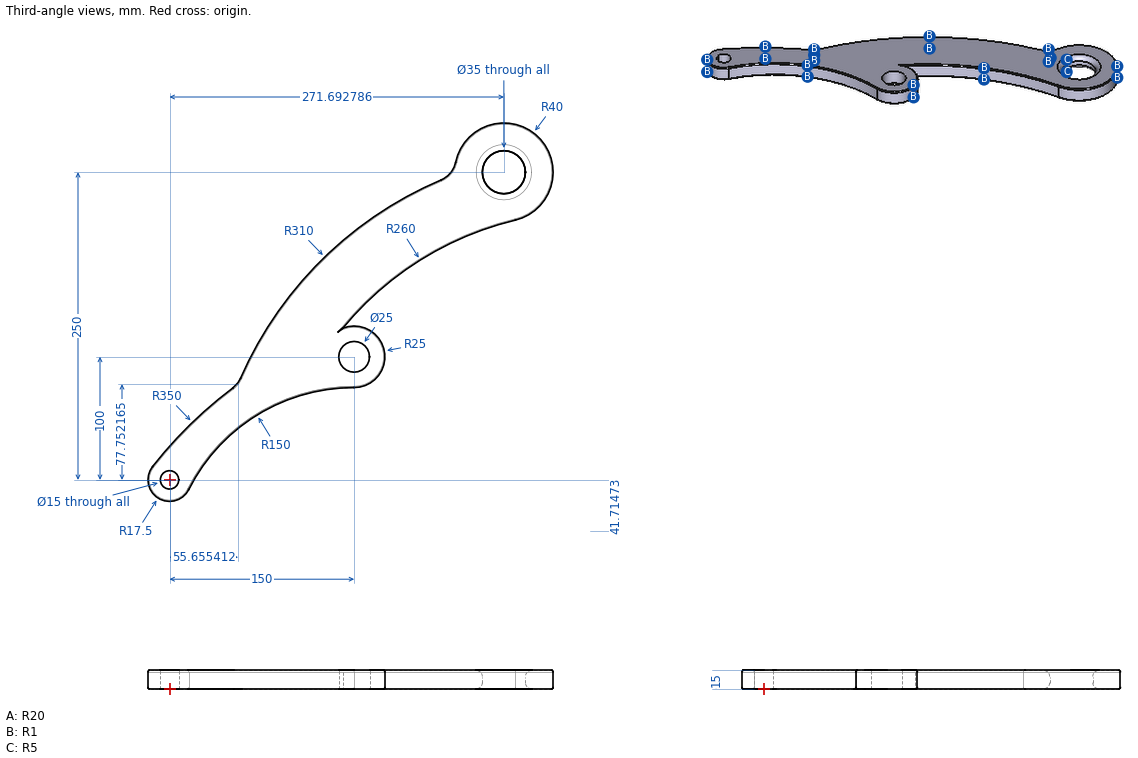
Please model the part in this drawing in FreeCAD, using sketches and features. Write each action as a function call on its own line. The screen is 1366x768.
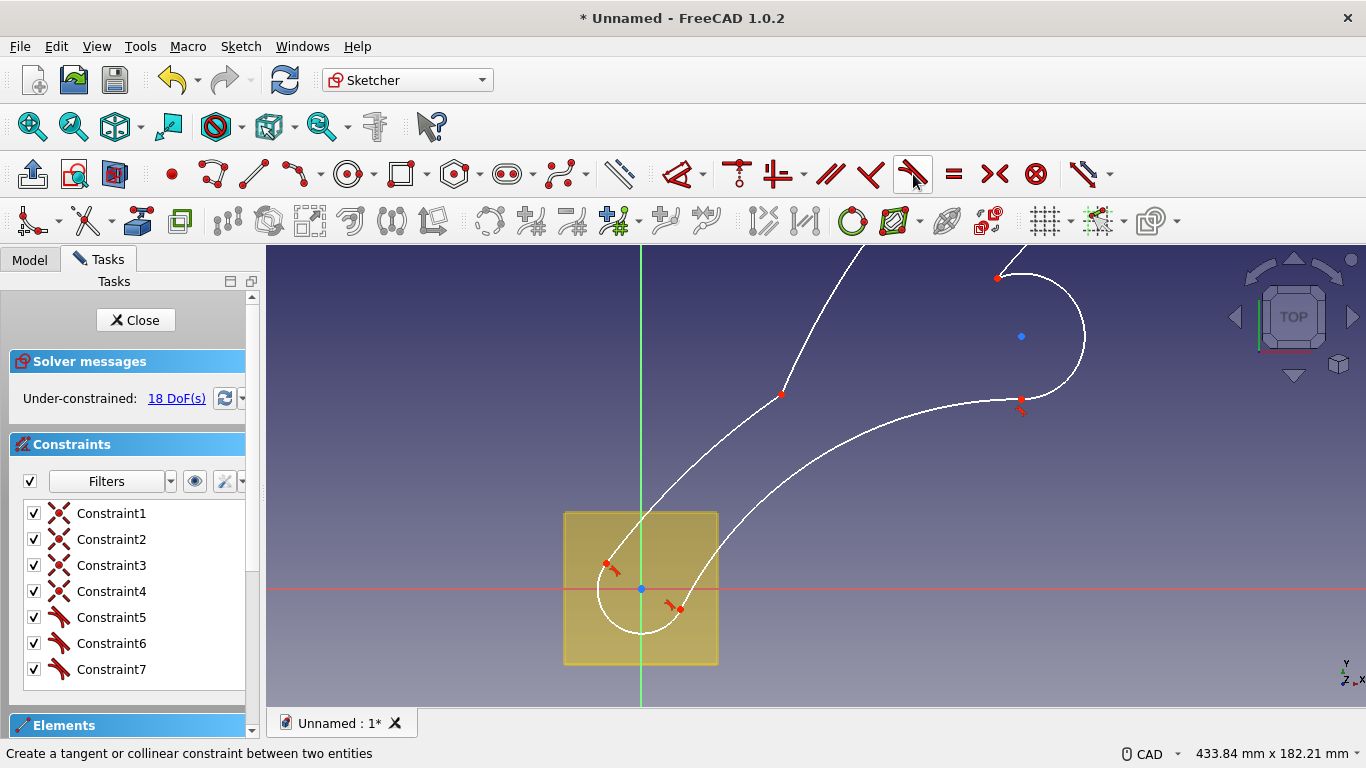
scroll(601, 608, down, 5)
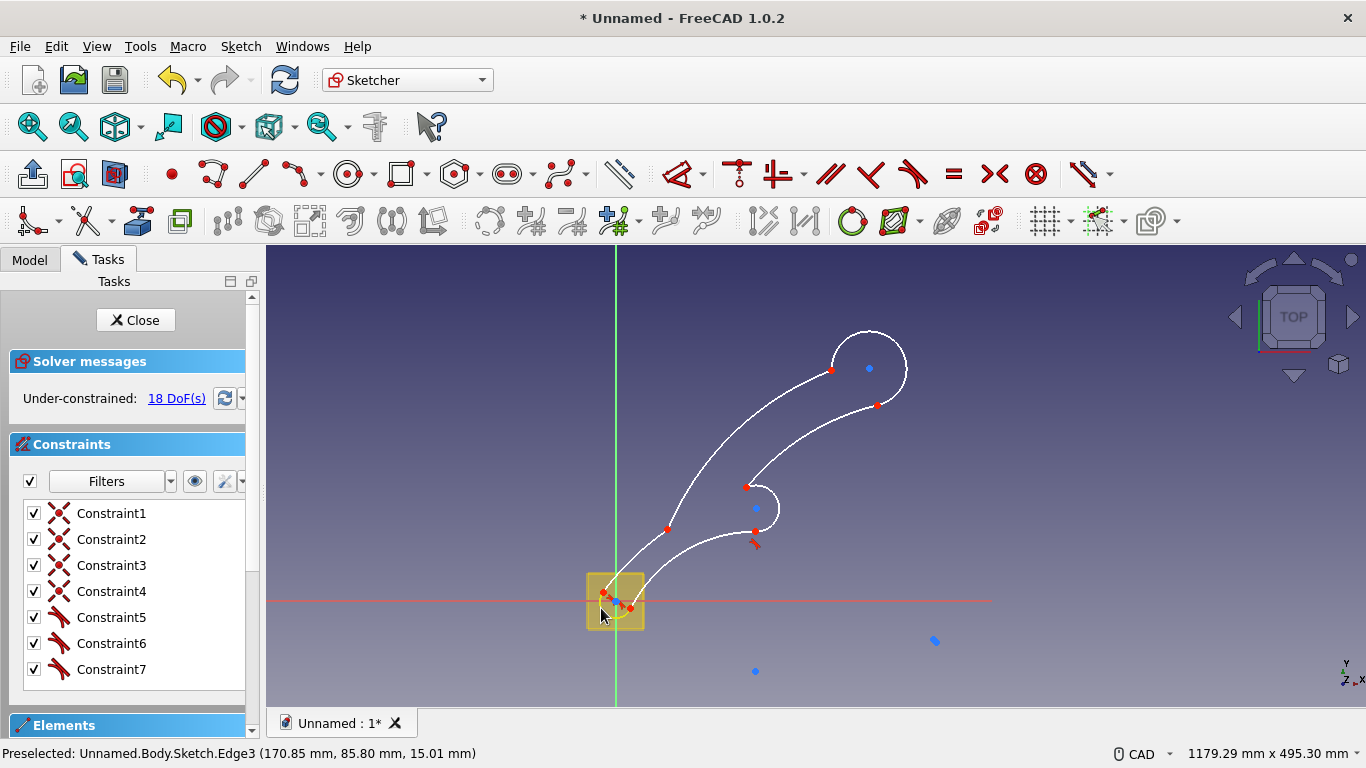
click(833, 421)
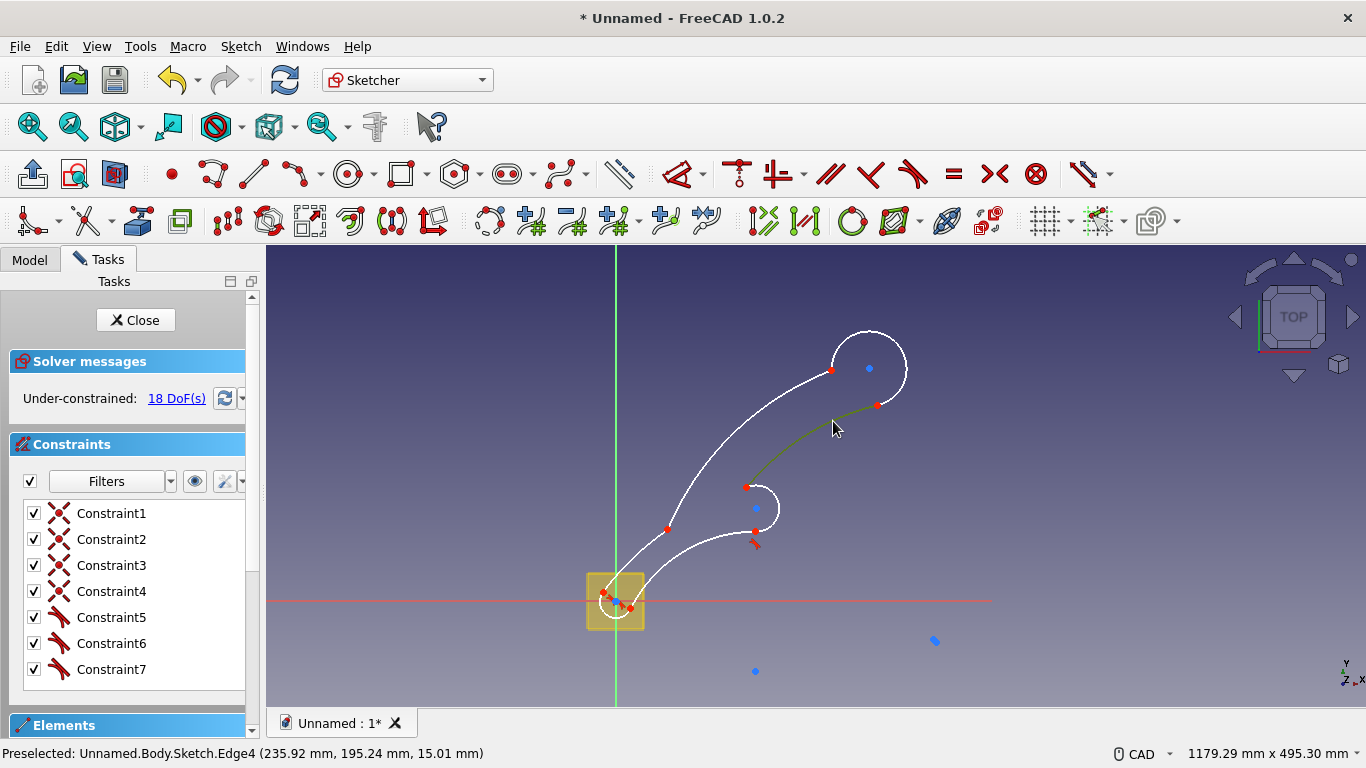
click(907, 368)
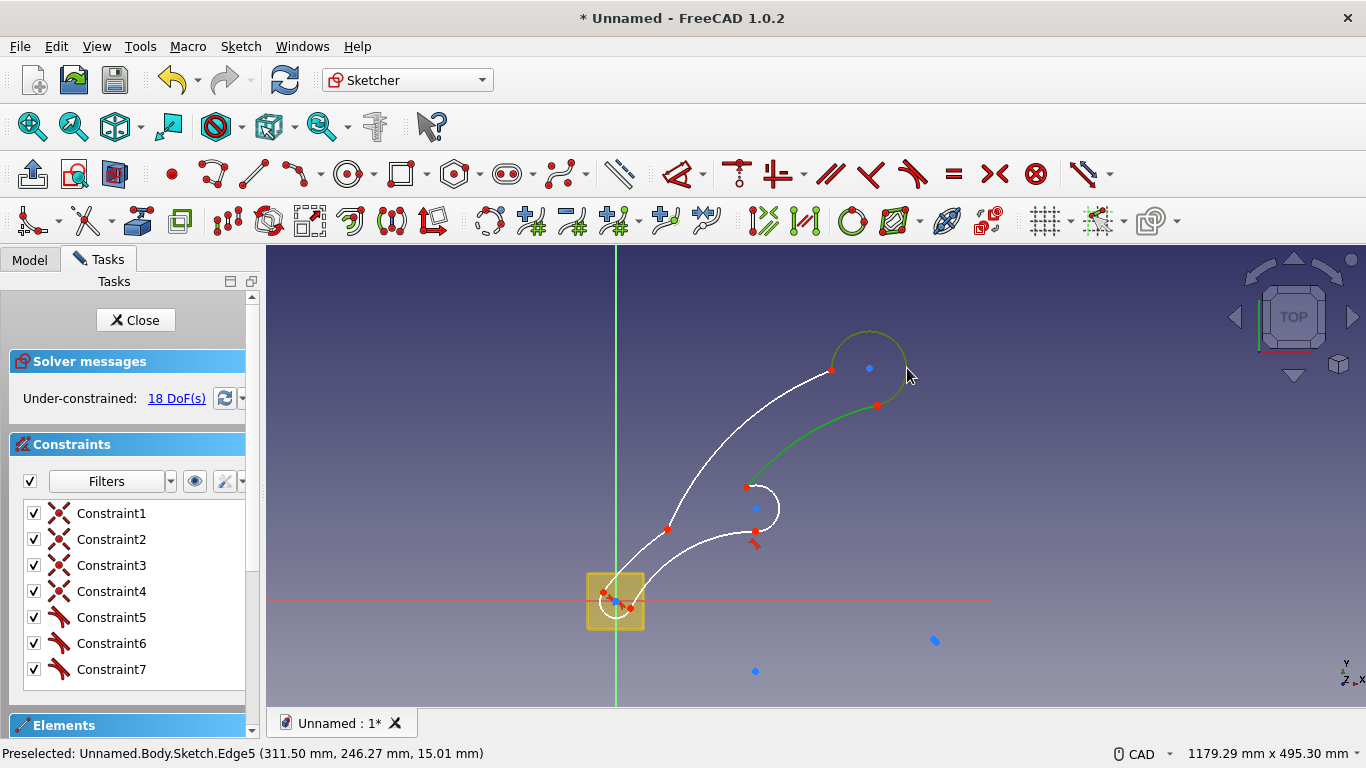
click(913, 174)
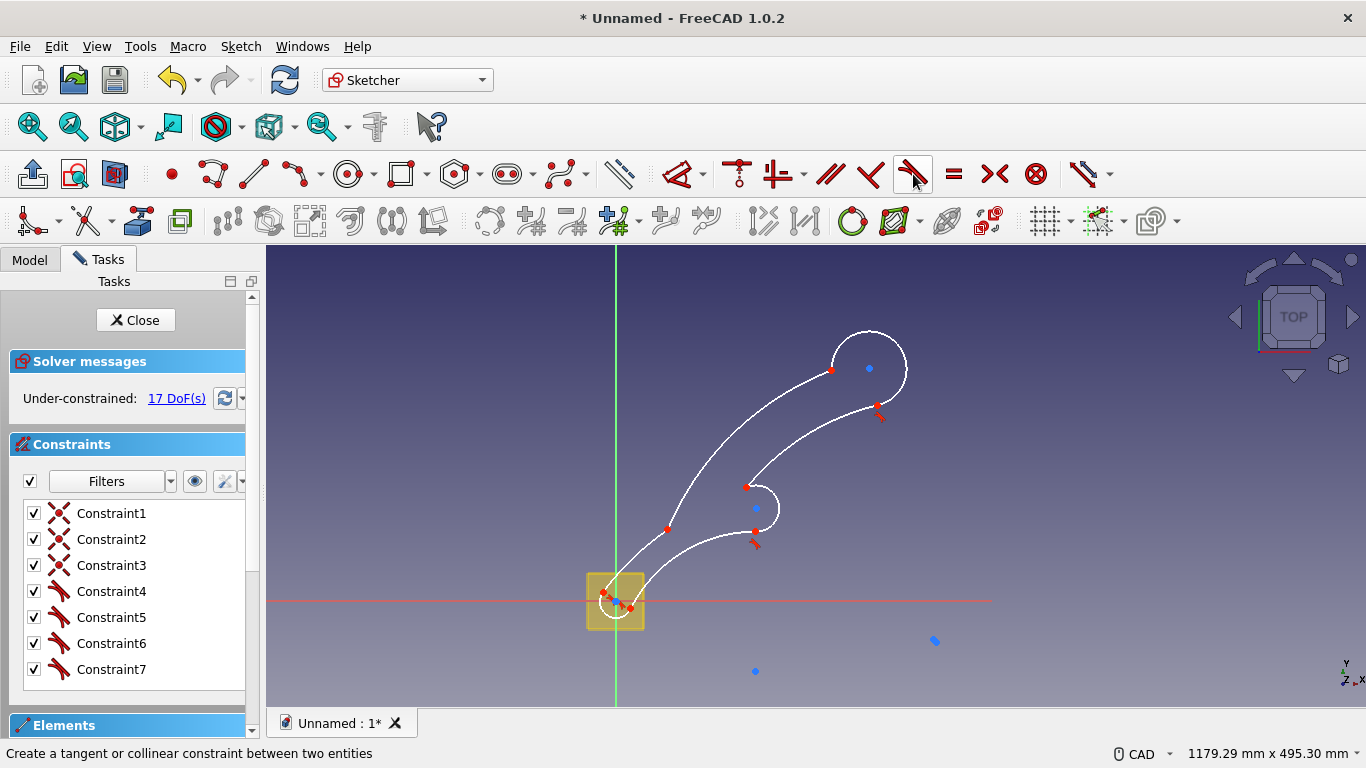
click(833, 421)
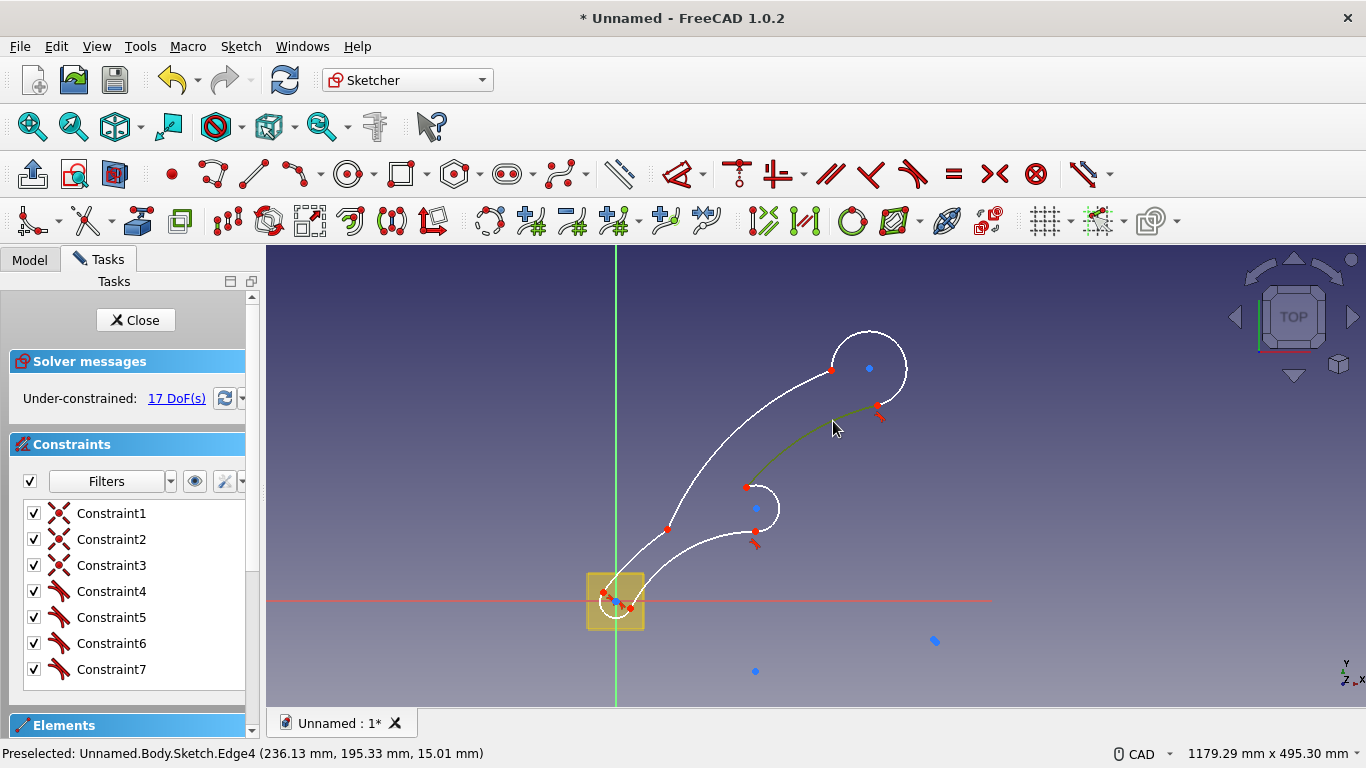
click(770, 403)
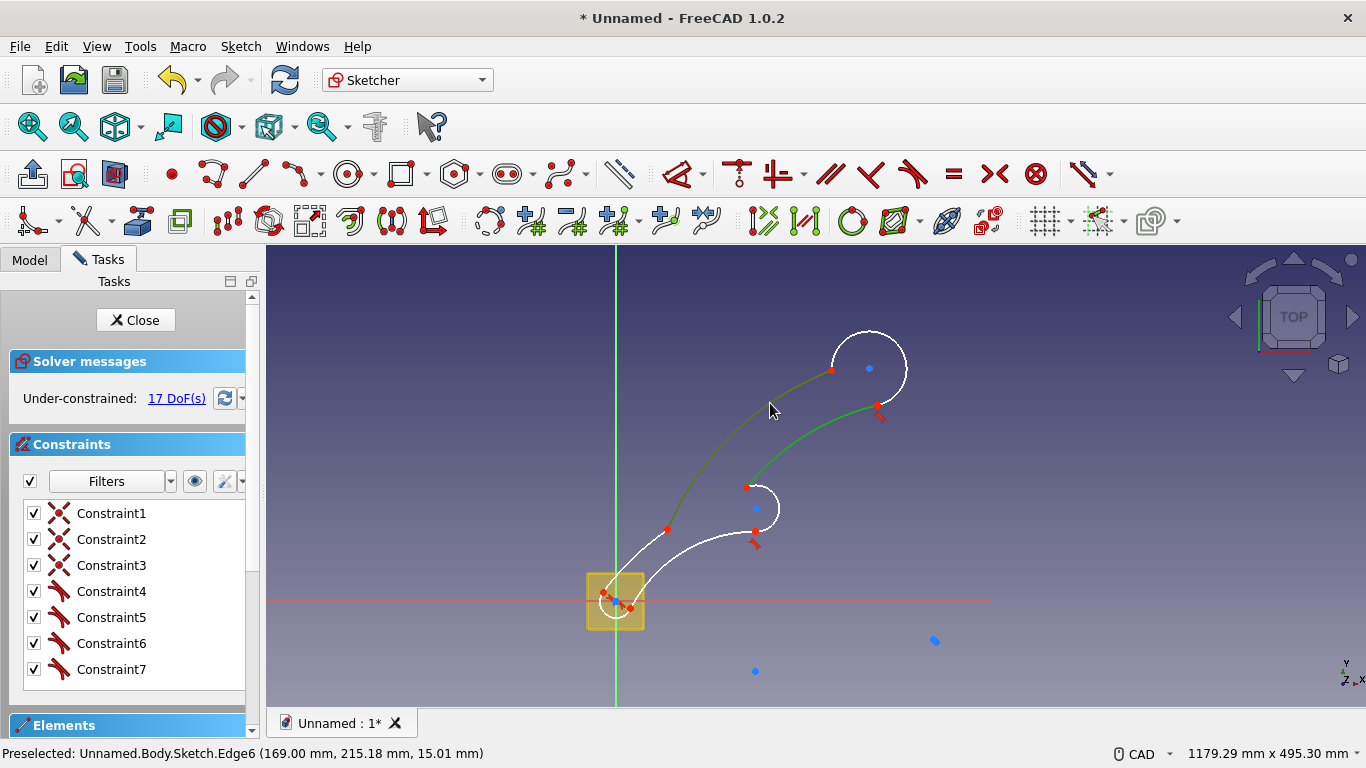
click(737, 174)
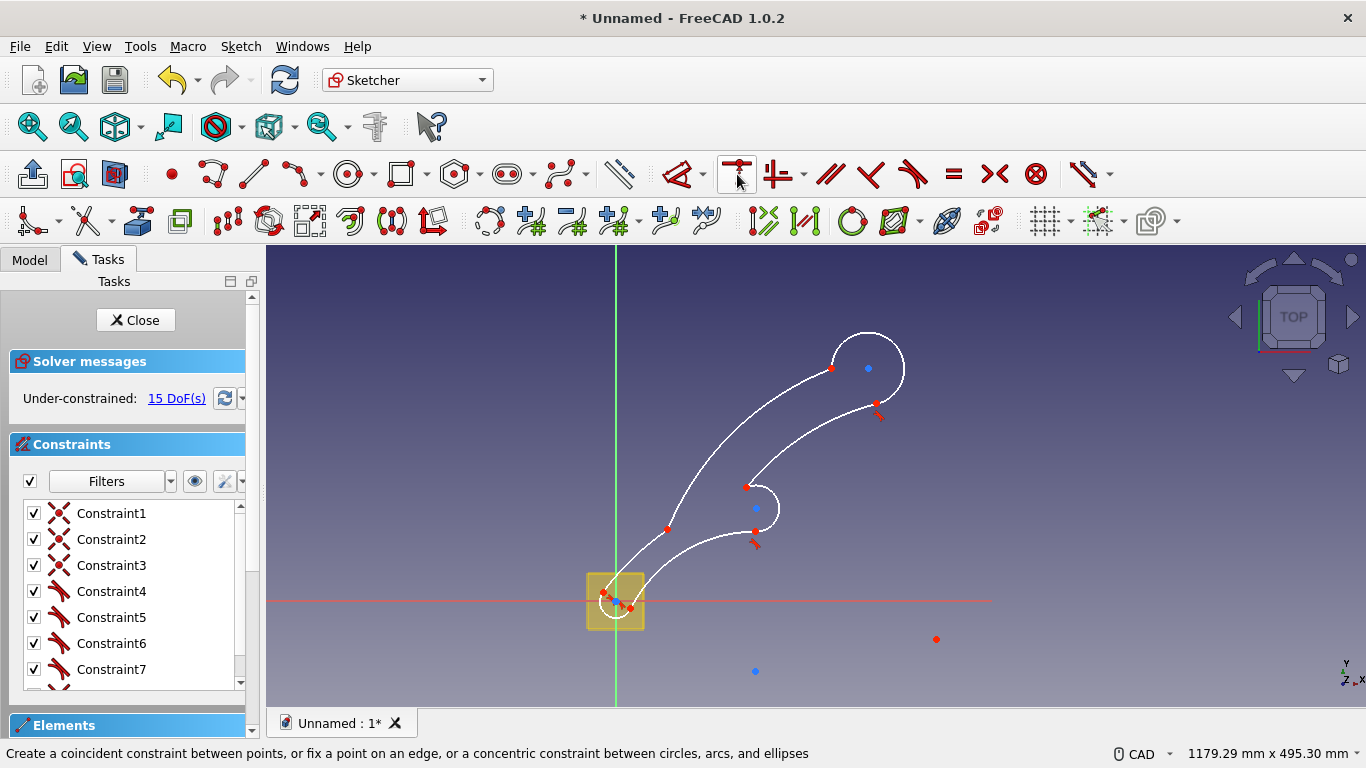
scroll(616, 602, up, 5)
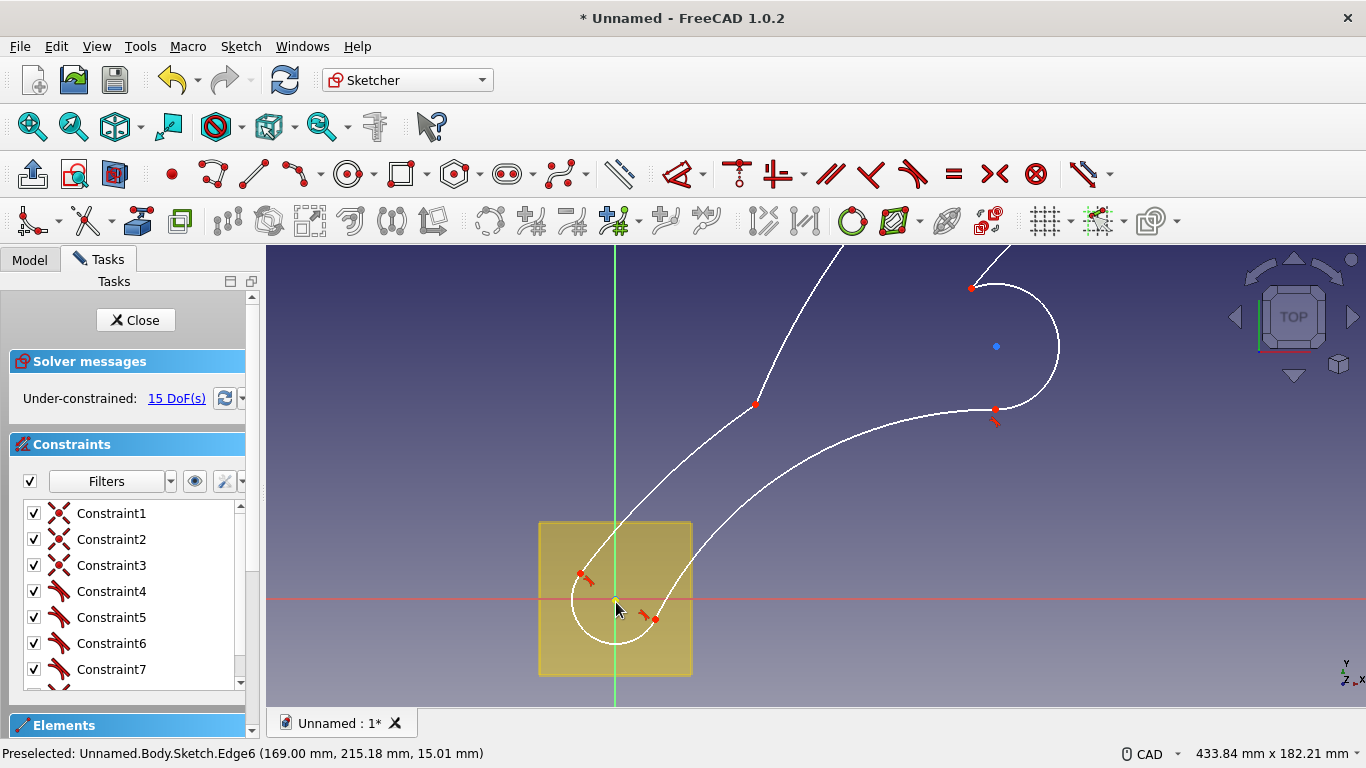
drag(605, 589, 626, 610)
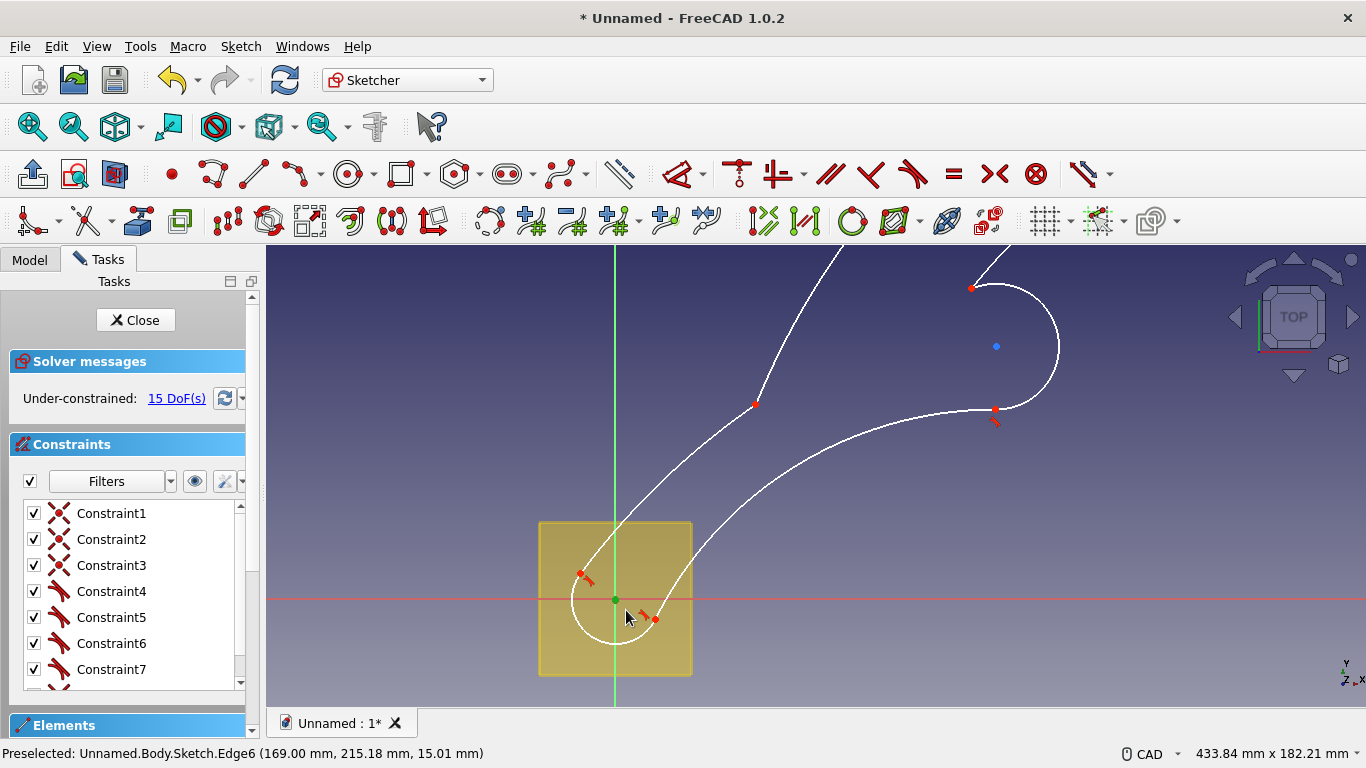
click(737, 174)